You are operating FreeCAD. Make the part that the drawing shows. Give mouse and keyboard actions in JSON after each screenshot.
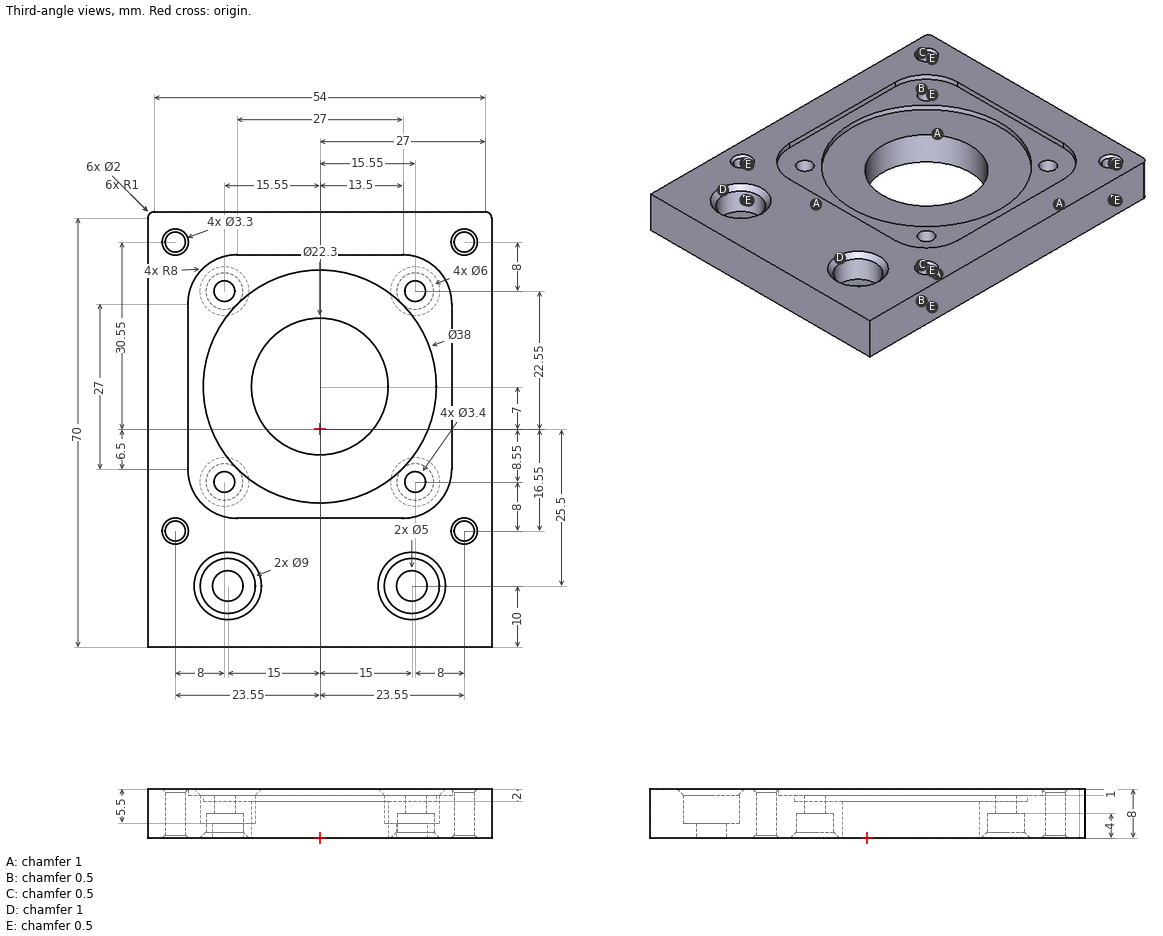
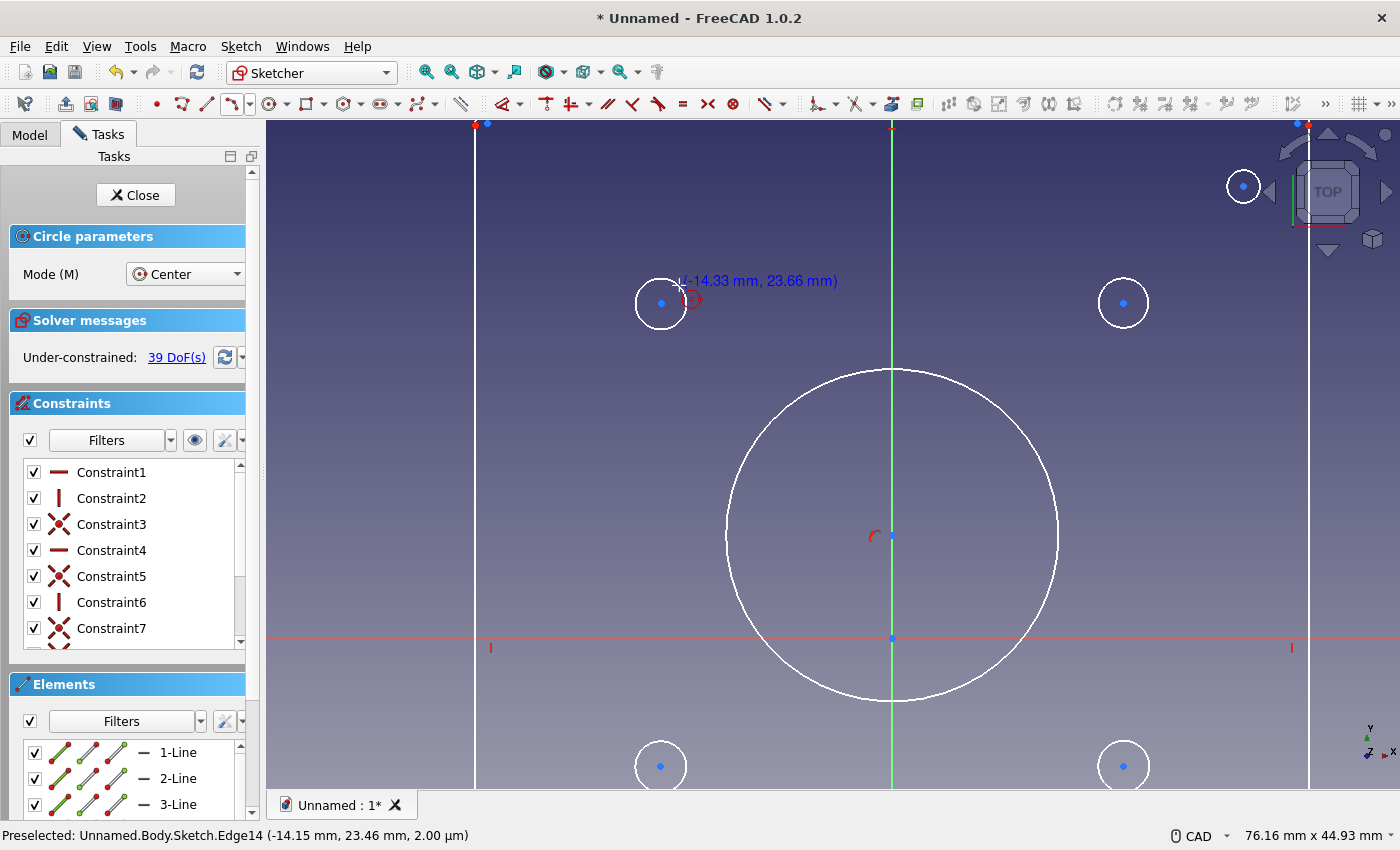
{"action": "scroll", "coordinate": [542, 183], "scroll_direction": "up", "scroll_amount": 3}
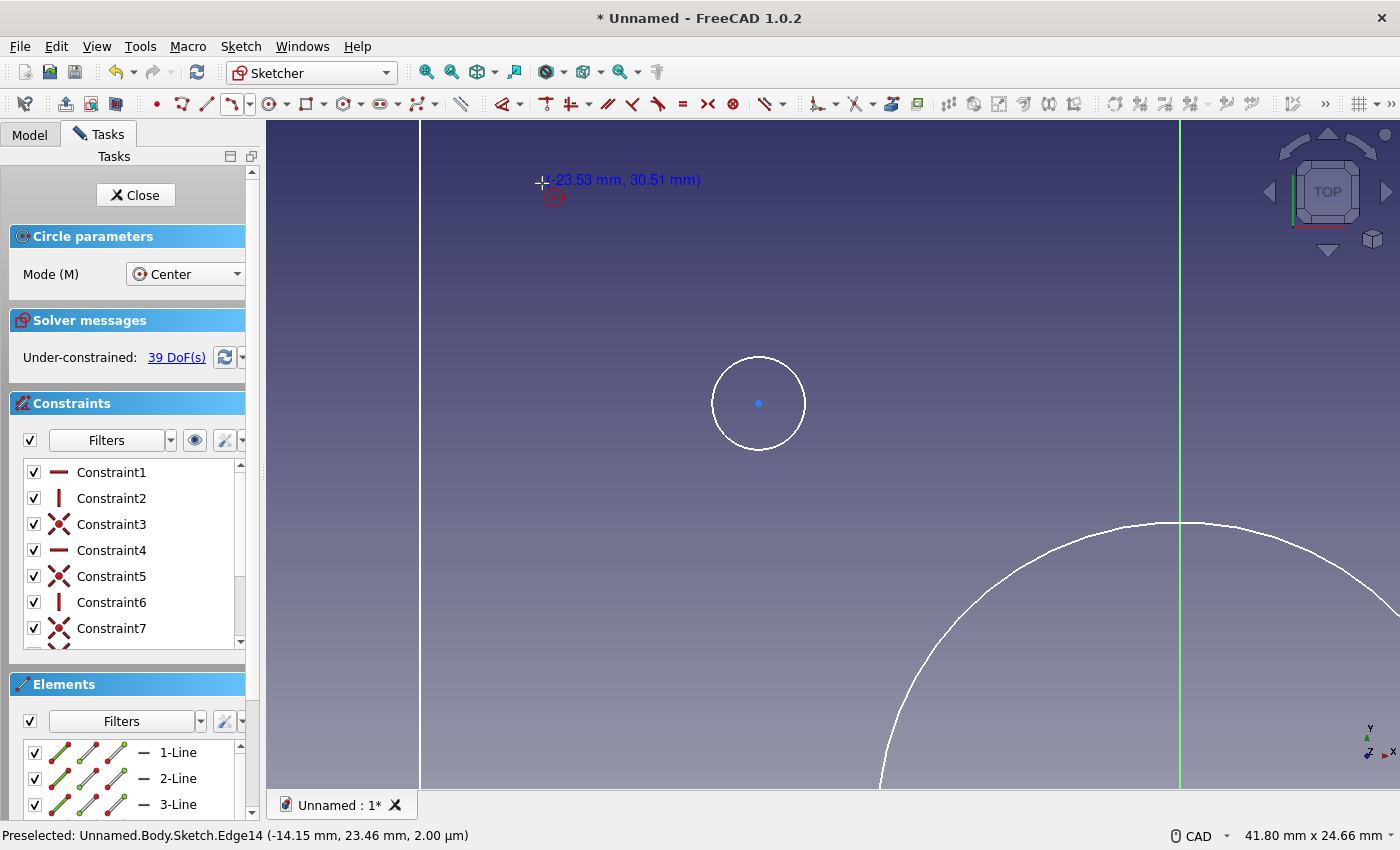
{"action": "scroll", "coordinate": [628, 272], "scroll_direction": "down", "scroll_amount": 7}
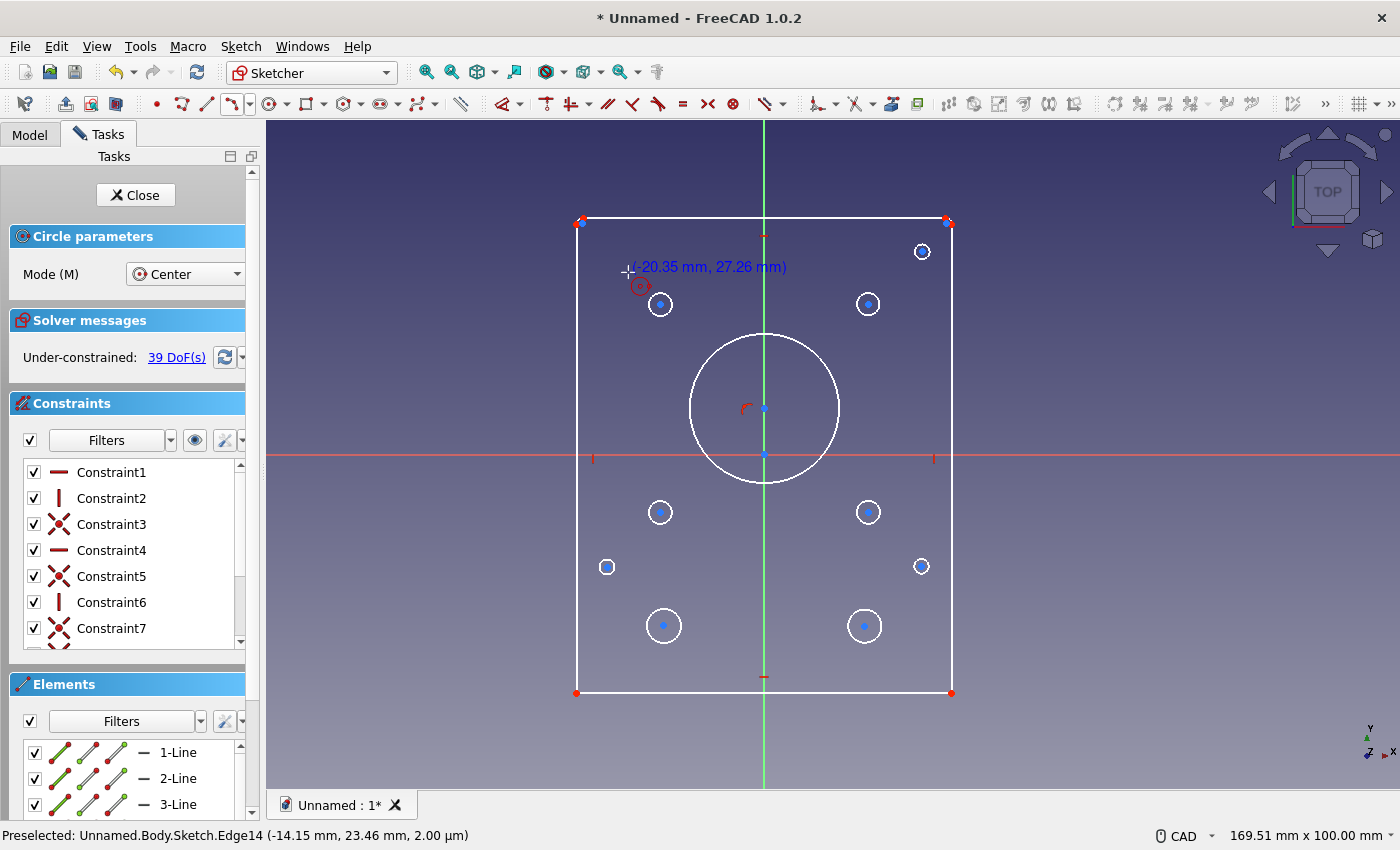
{"action": "left_click", "coordinate": [607, 250]}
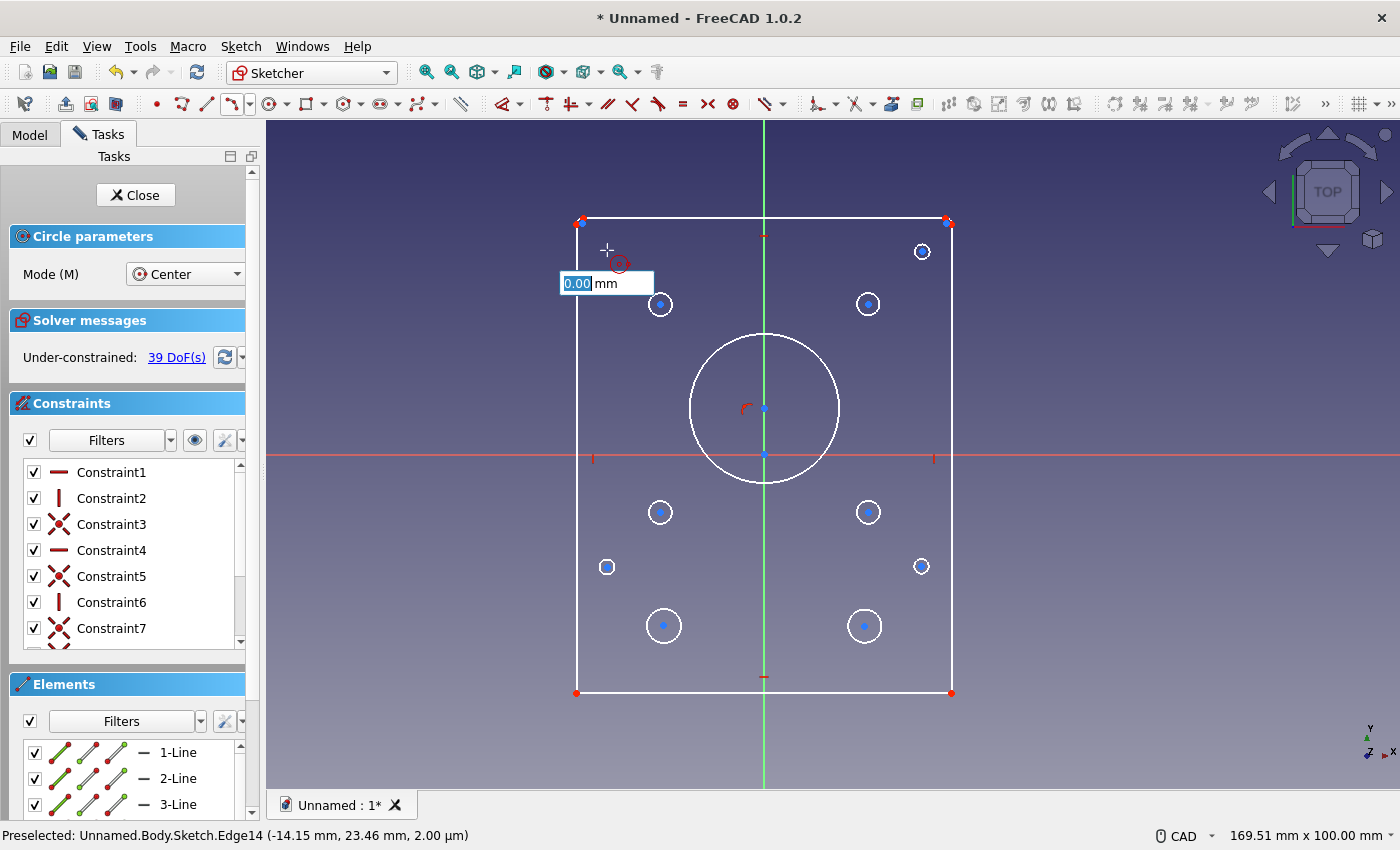
{"action": "scroll", "coordinate": [612, 246], "scroll_direction": "up", "scroll_amount": 5}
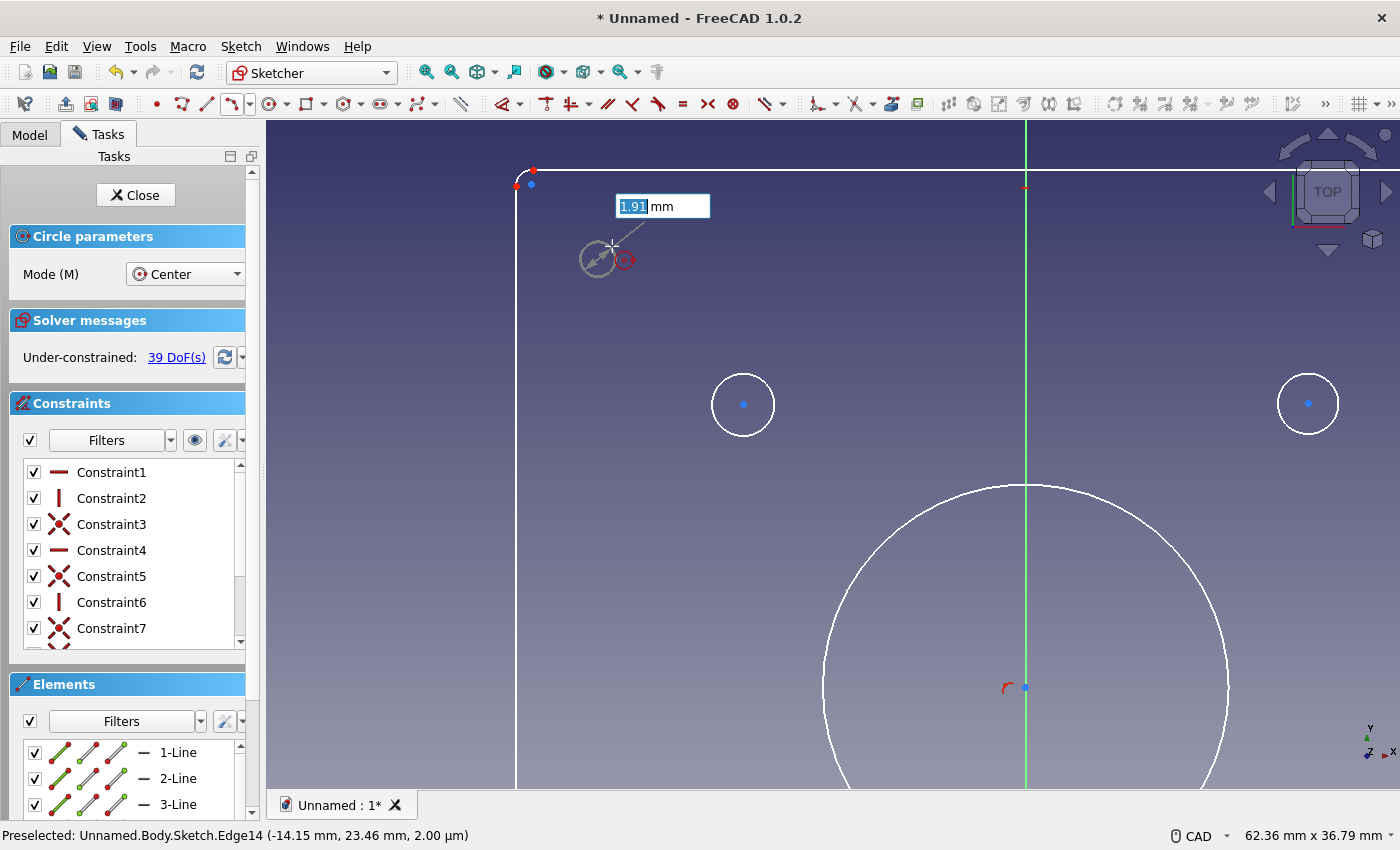
{"action": "left_click", "coordinate": [610, 245]}
{"action": "key", "text": "Escape"}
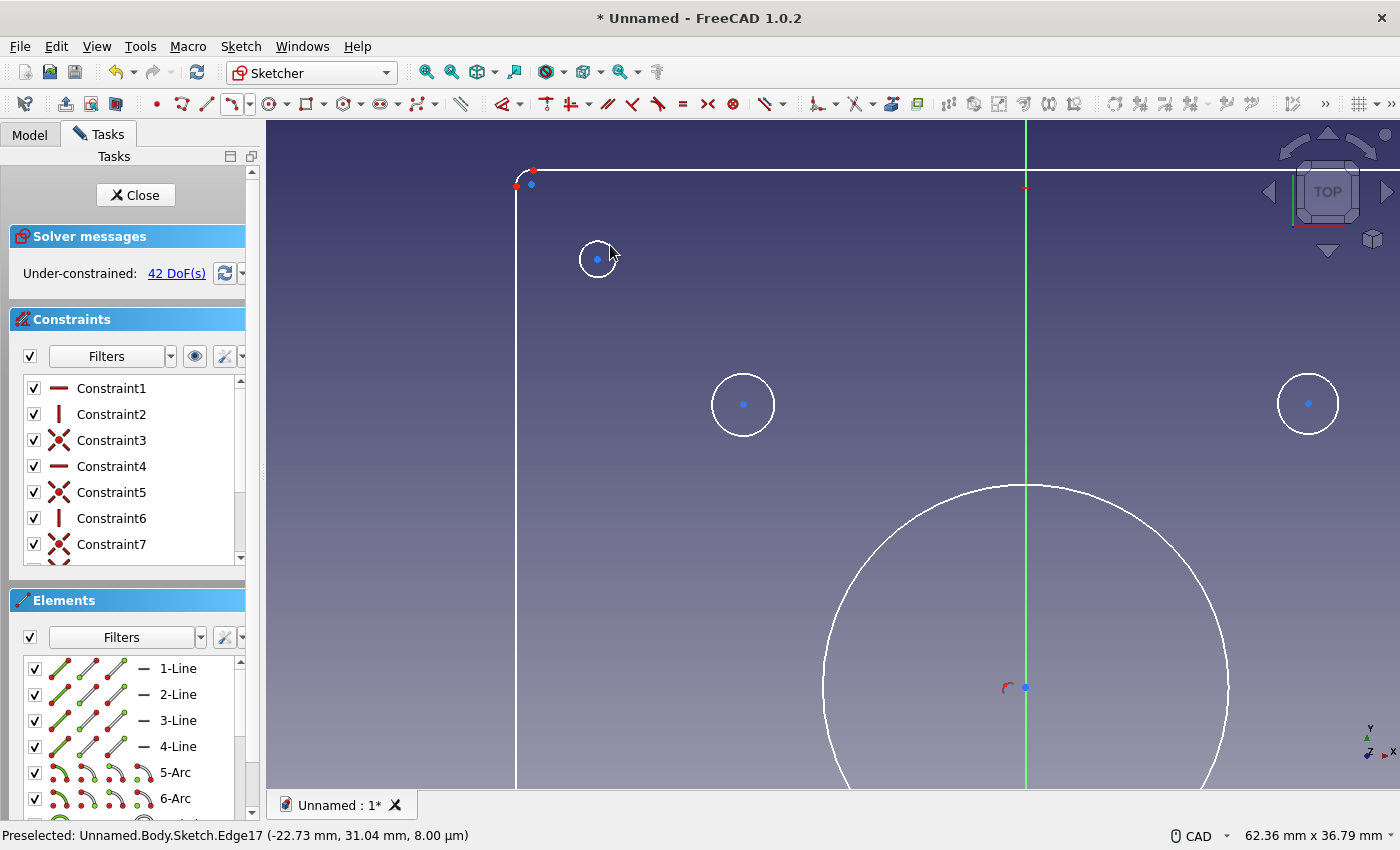
{"action": "left_click", "coordinate": [1223, 170]}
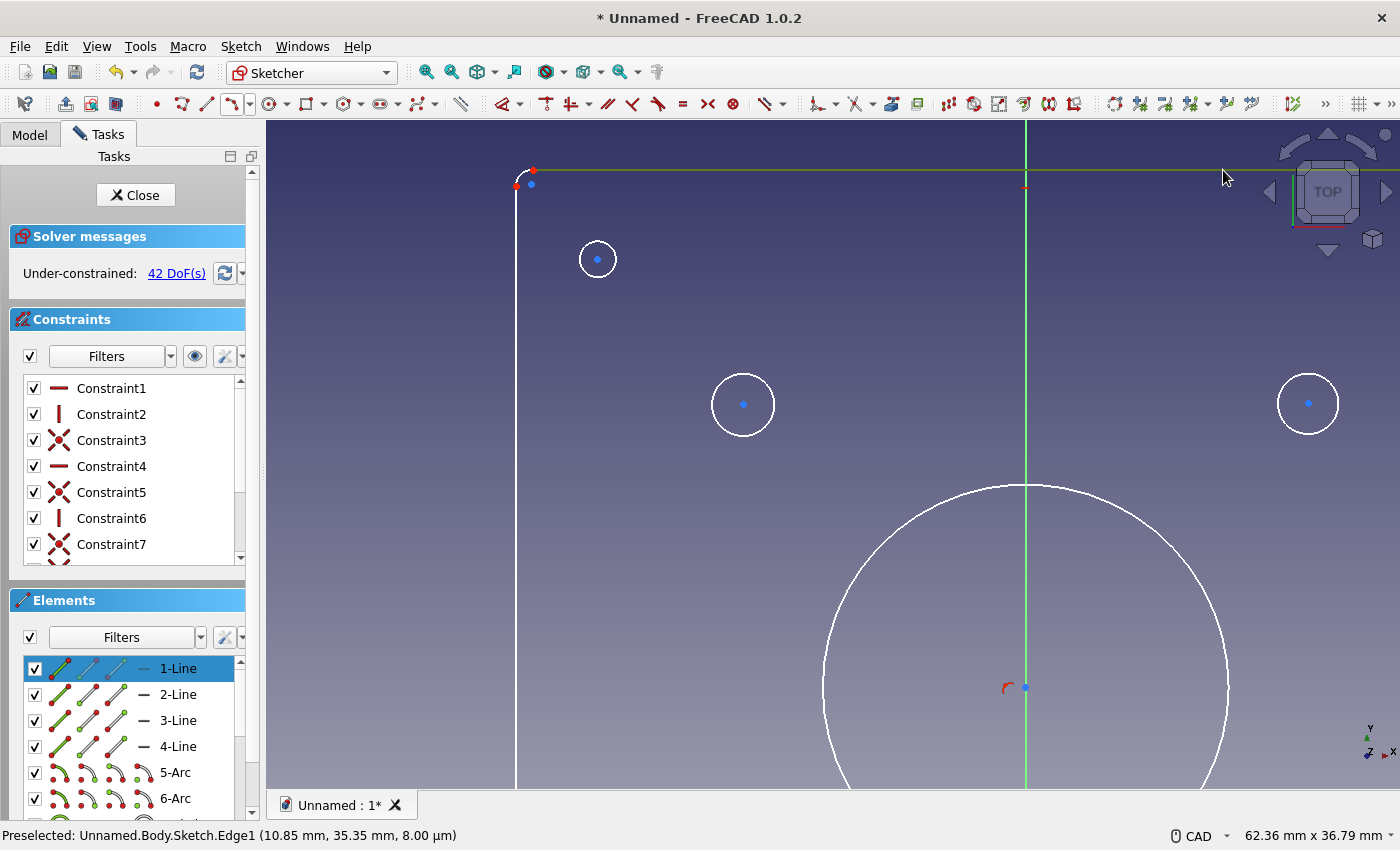
{"action": "left_click", "coordinate": [521, 174]}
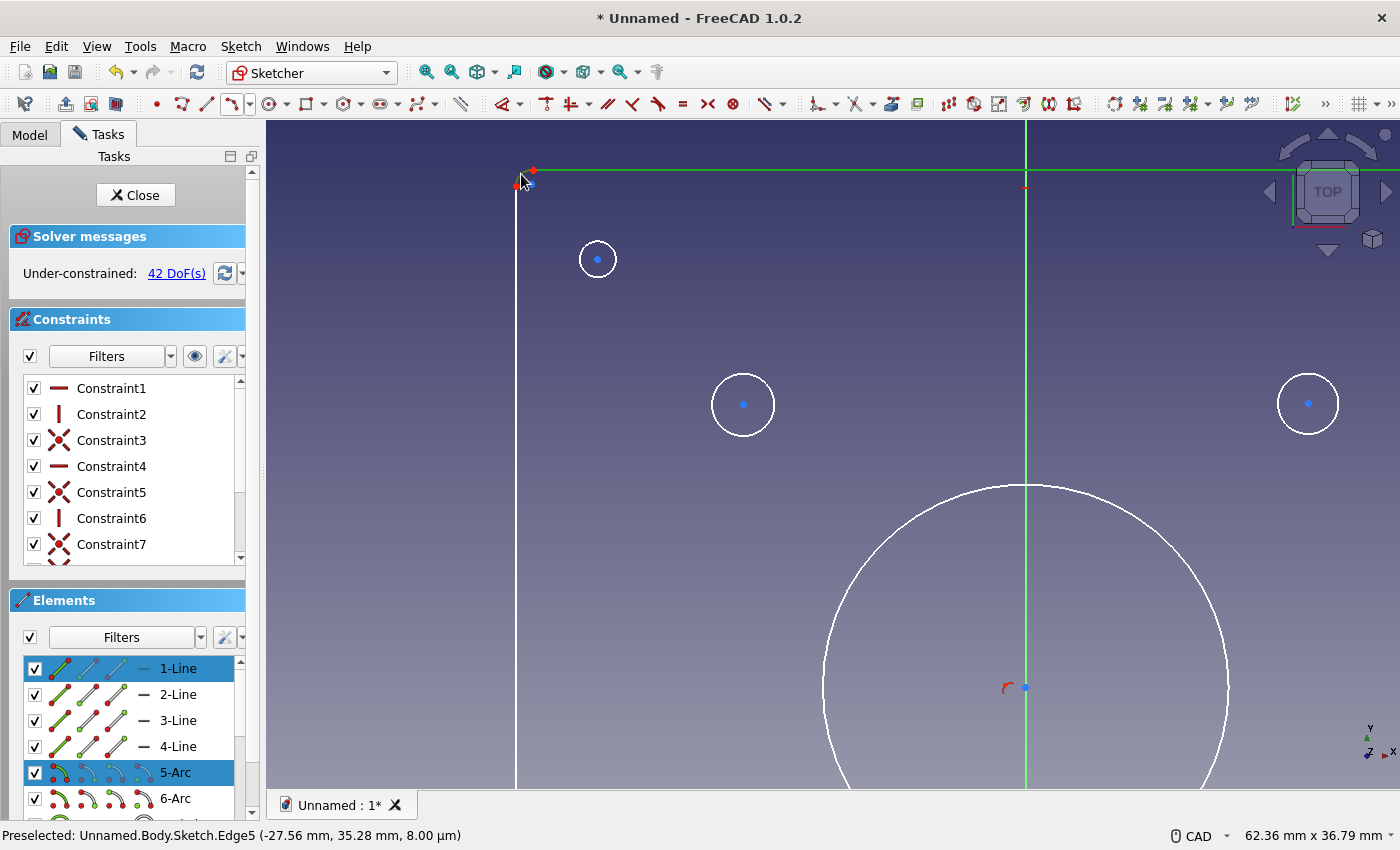
{"action": "key", "text": "t"}